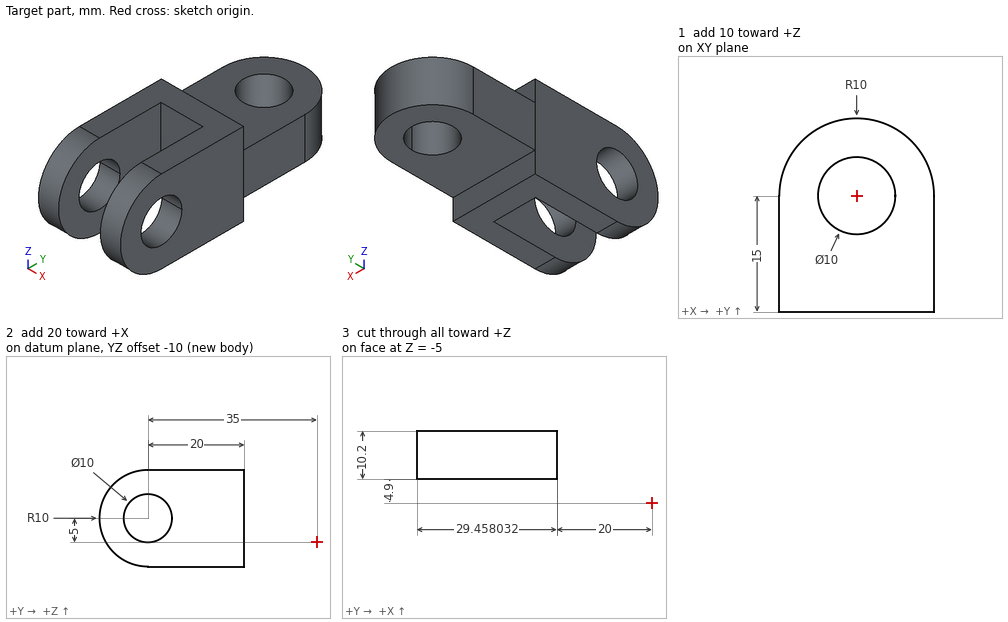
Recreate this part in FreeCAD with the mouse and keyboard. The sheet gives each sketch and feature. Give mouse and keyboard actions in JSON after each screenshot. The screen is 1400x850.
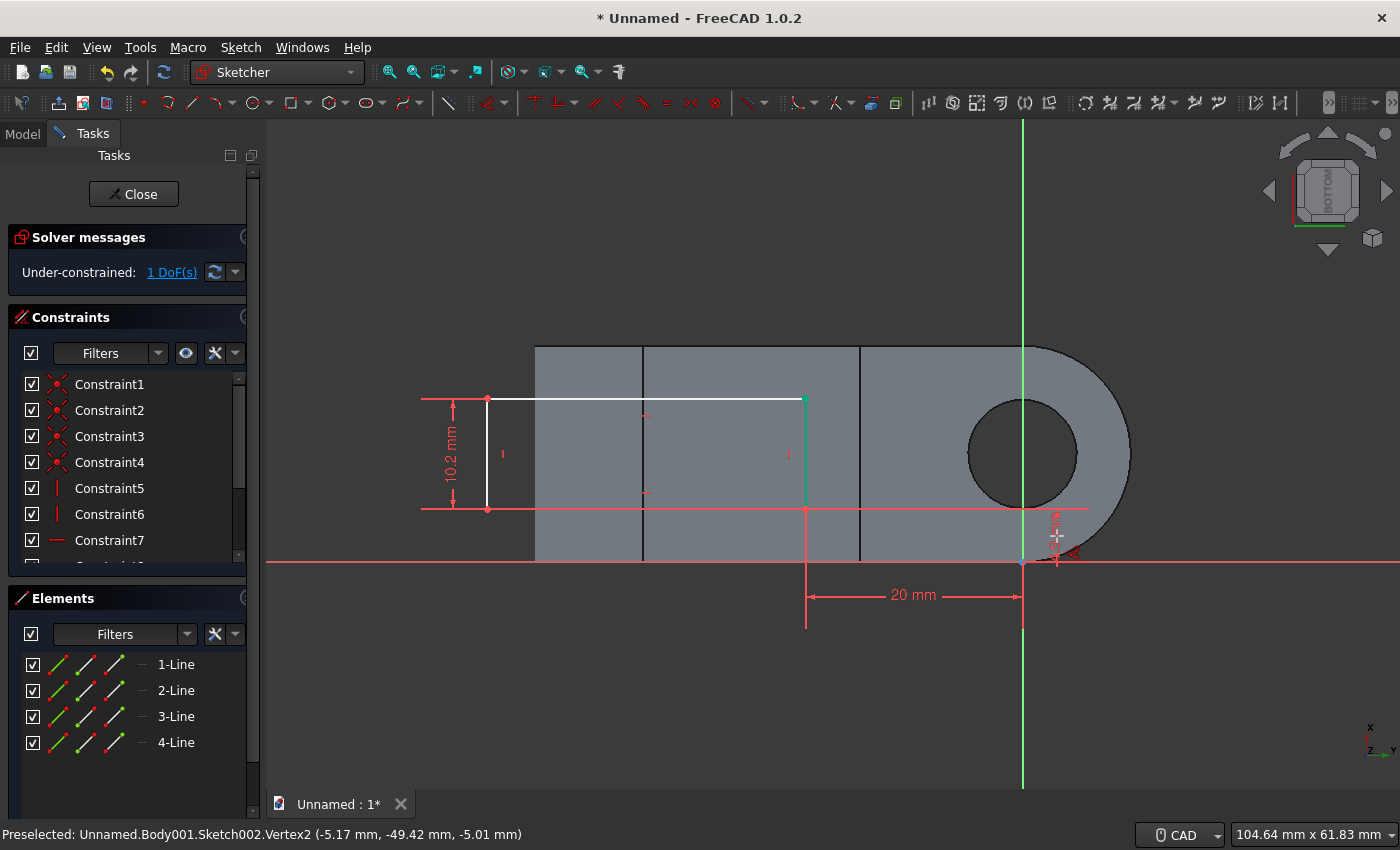
{"action": "left_click", "coordinate": [583, 509]}
{"action": "left_click", "coordinate": [646, 543]}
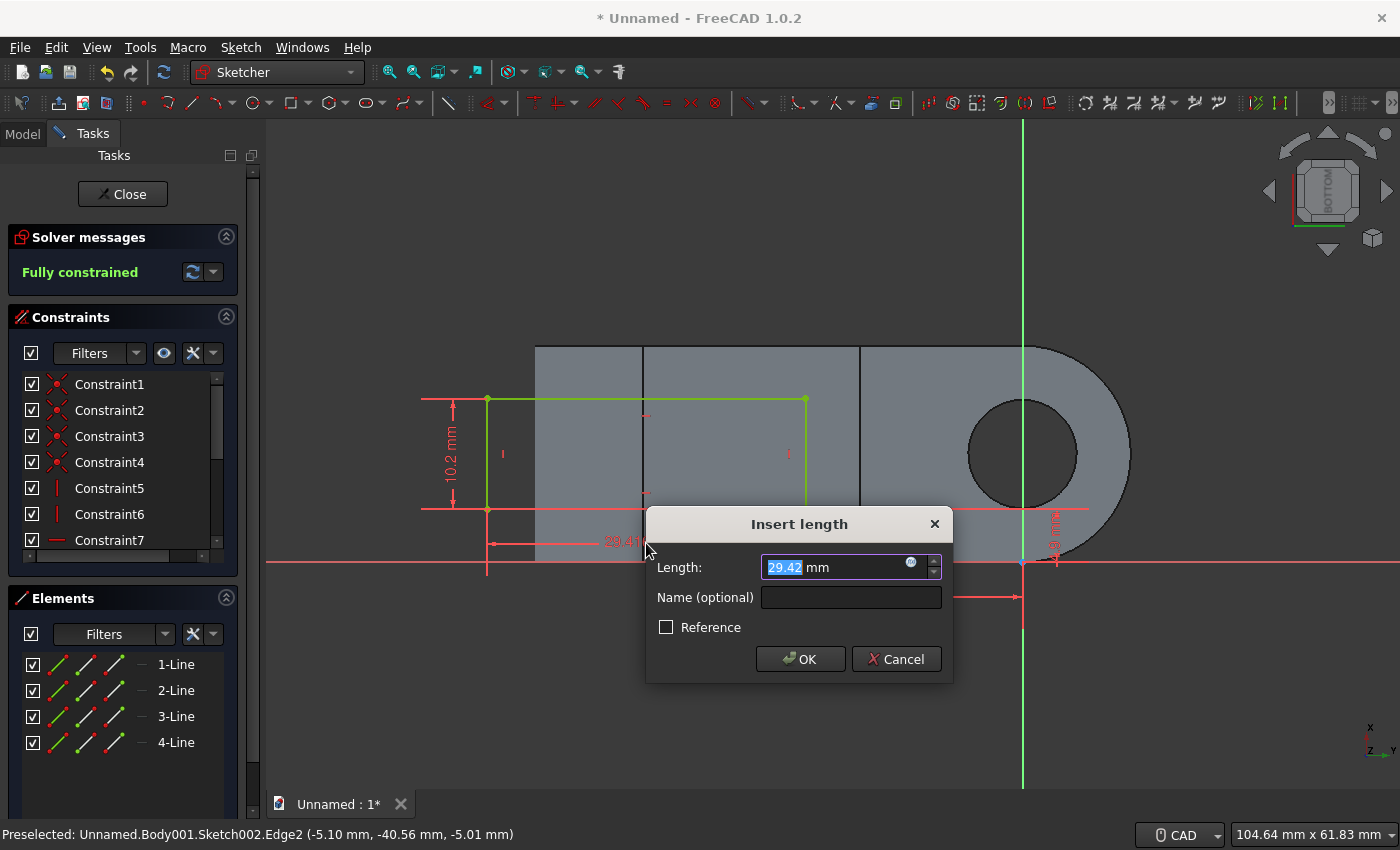
{"action": "type", "text": "29.458032"}
{"action": "key", "text": "Return"}
{"action": "key", "text": "Escape"}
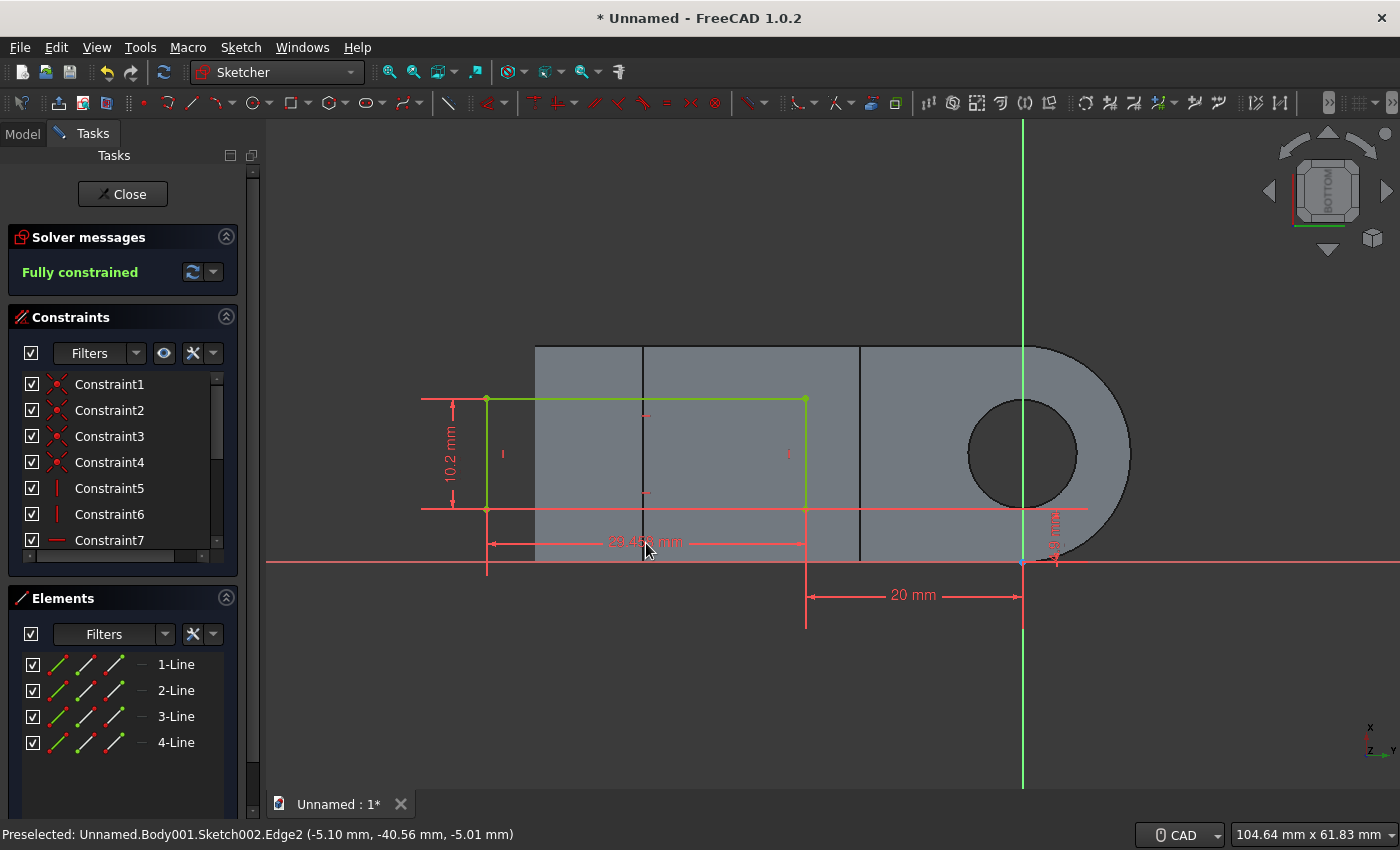
{"action": "left_click", "coordinate": [123, 194]}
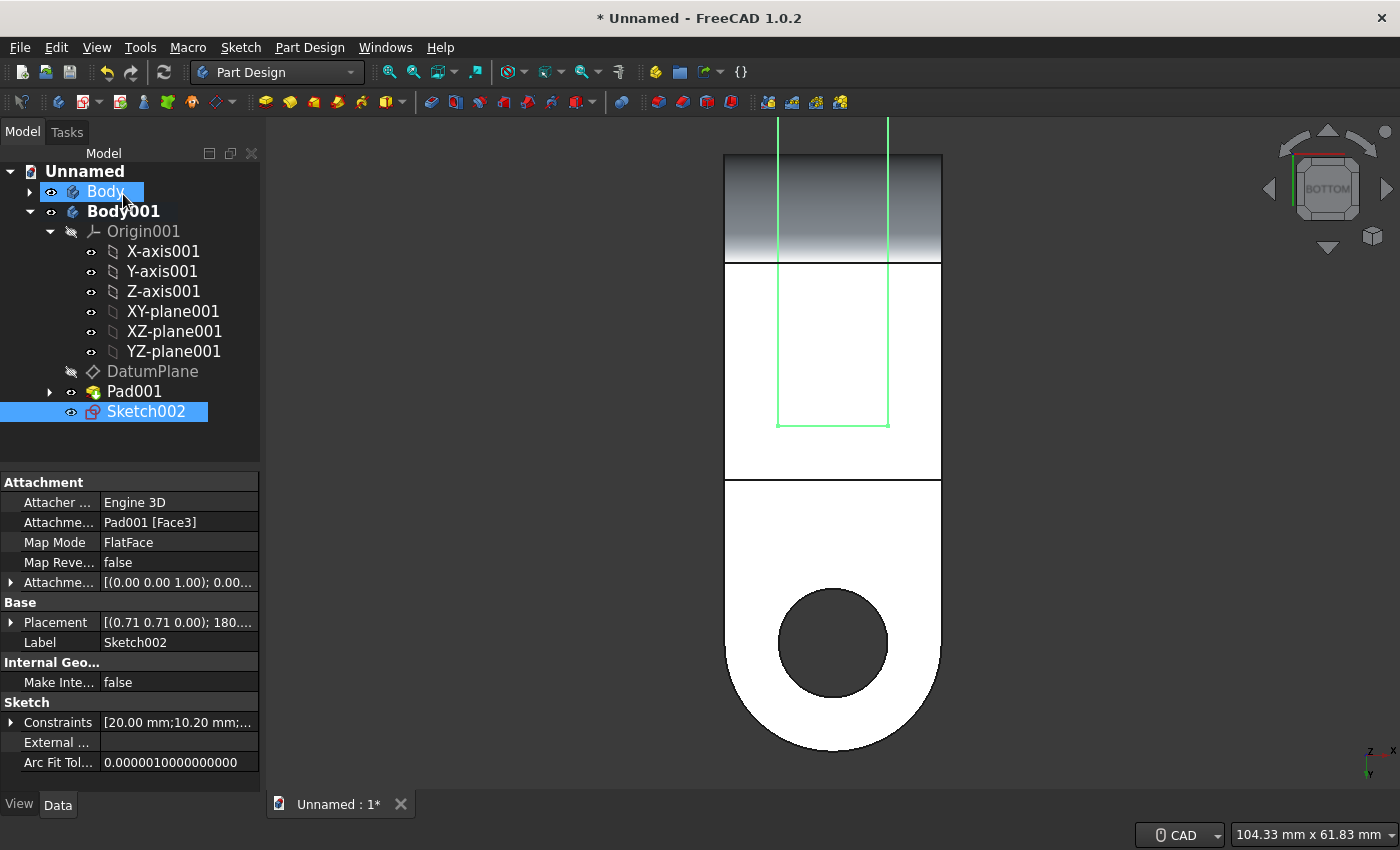
{"action": "left_click", "coordinate": [432, 102]}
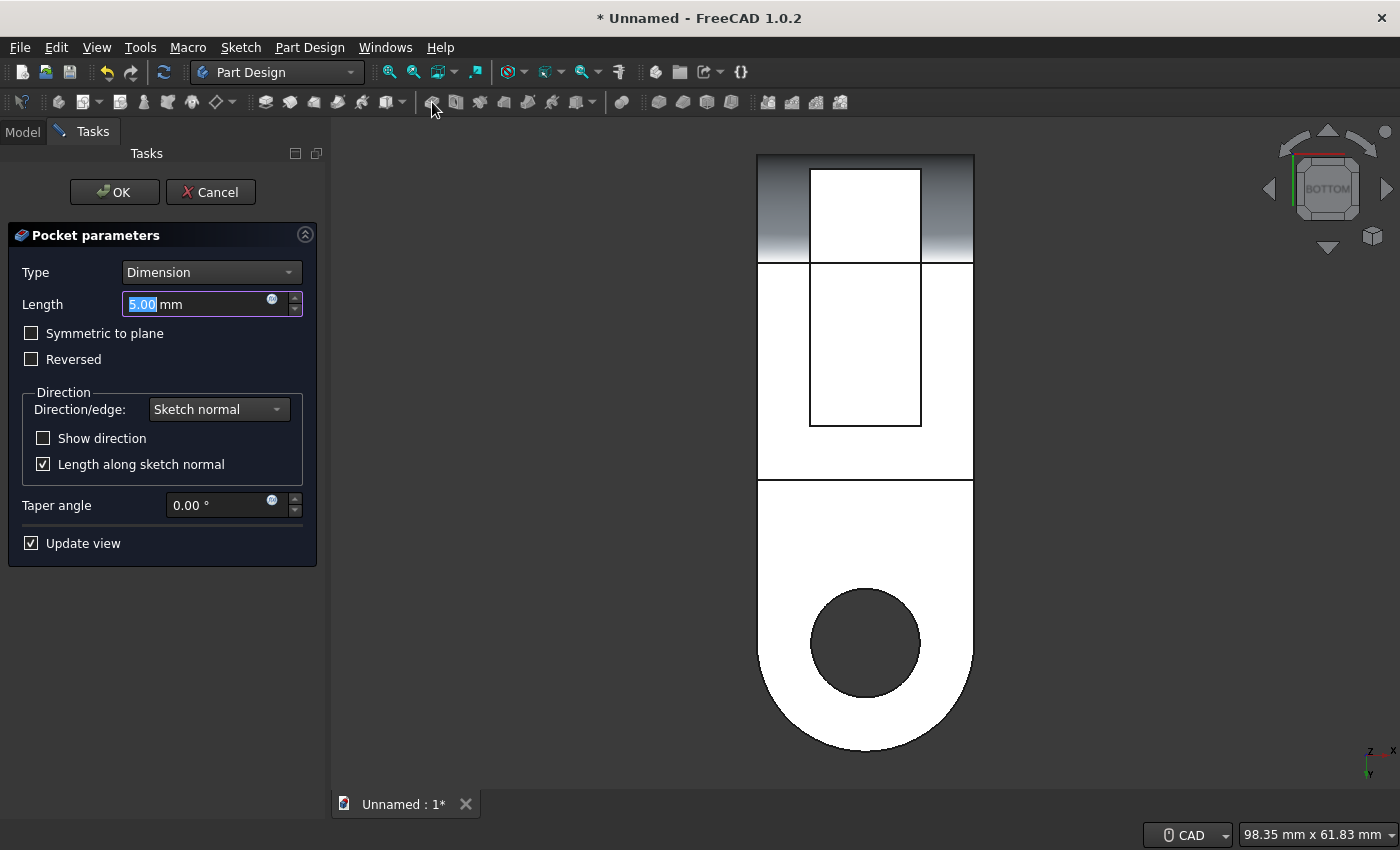
{"action": "left_click", "coordinate": [212, 272]}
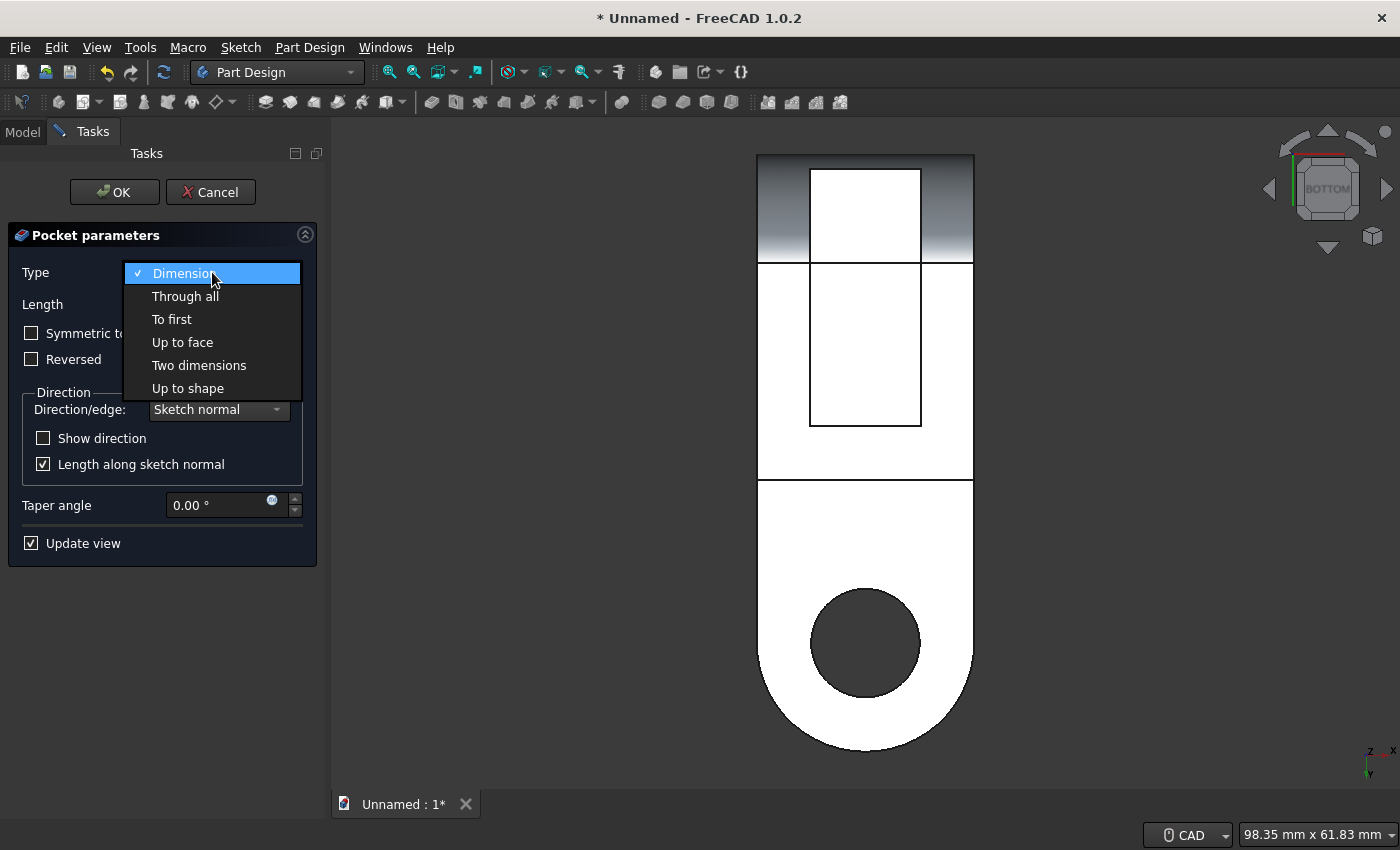
{"action": "left_click", "coordinate": [212, 296]}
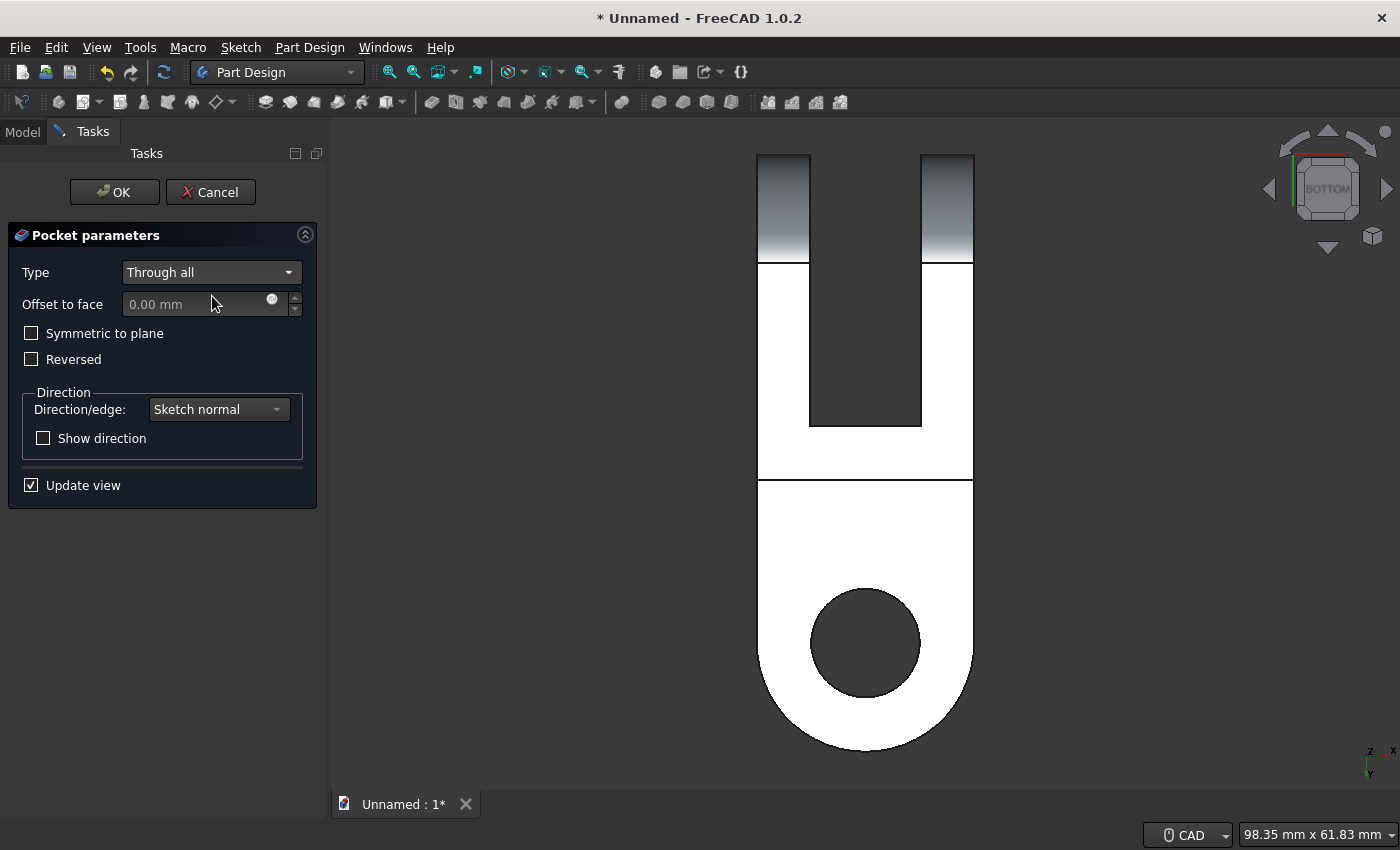
{"action": "left_click", "coordinate": [115, 192]}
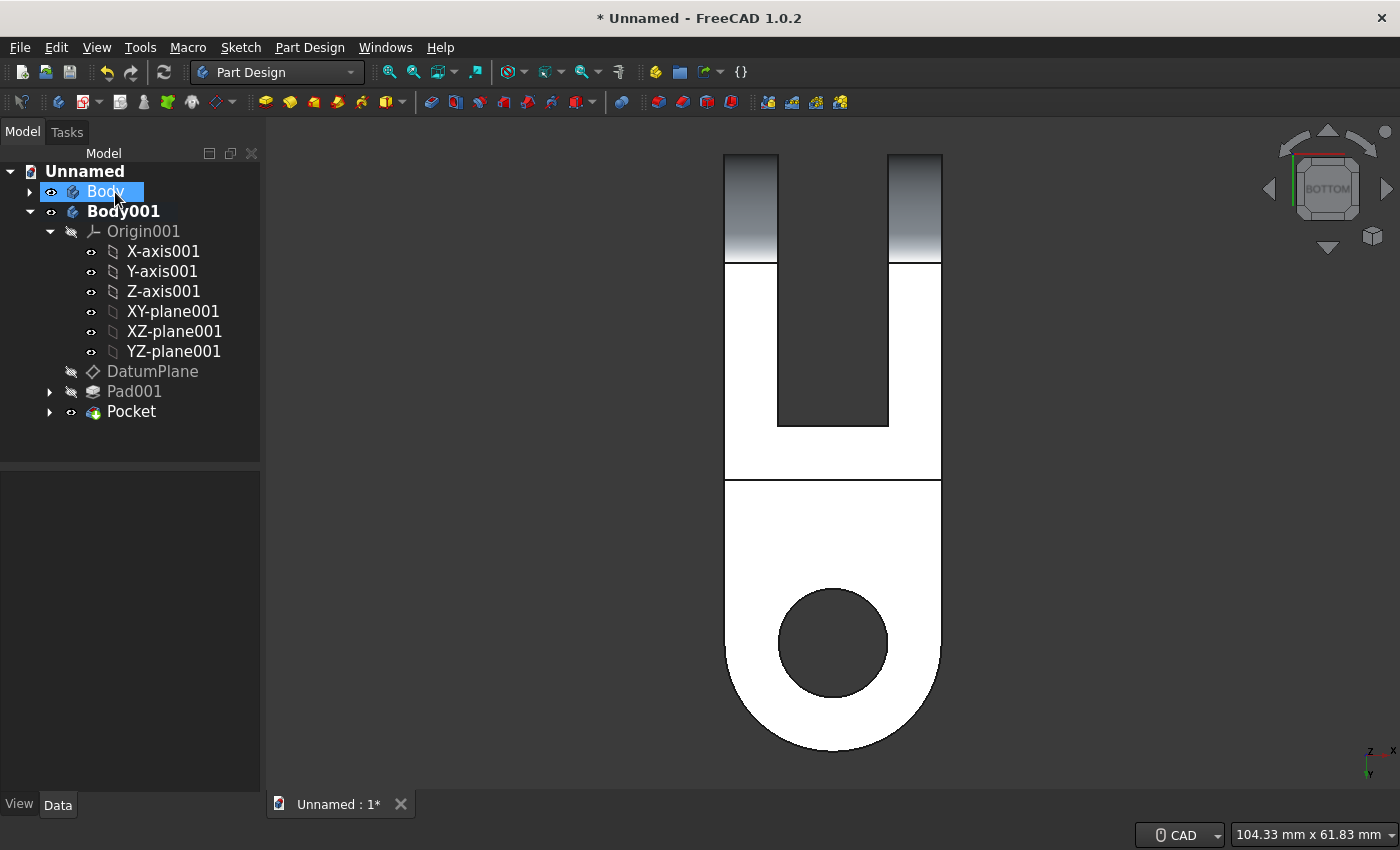
{"action": "key", "text": "0"}